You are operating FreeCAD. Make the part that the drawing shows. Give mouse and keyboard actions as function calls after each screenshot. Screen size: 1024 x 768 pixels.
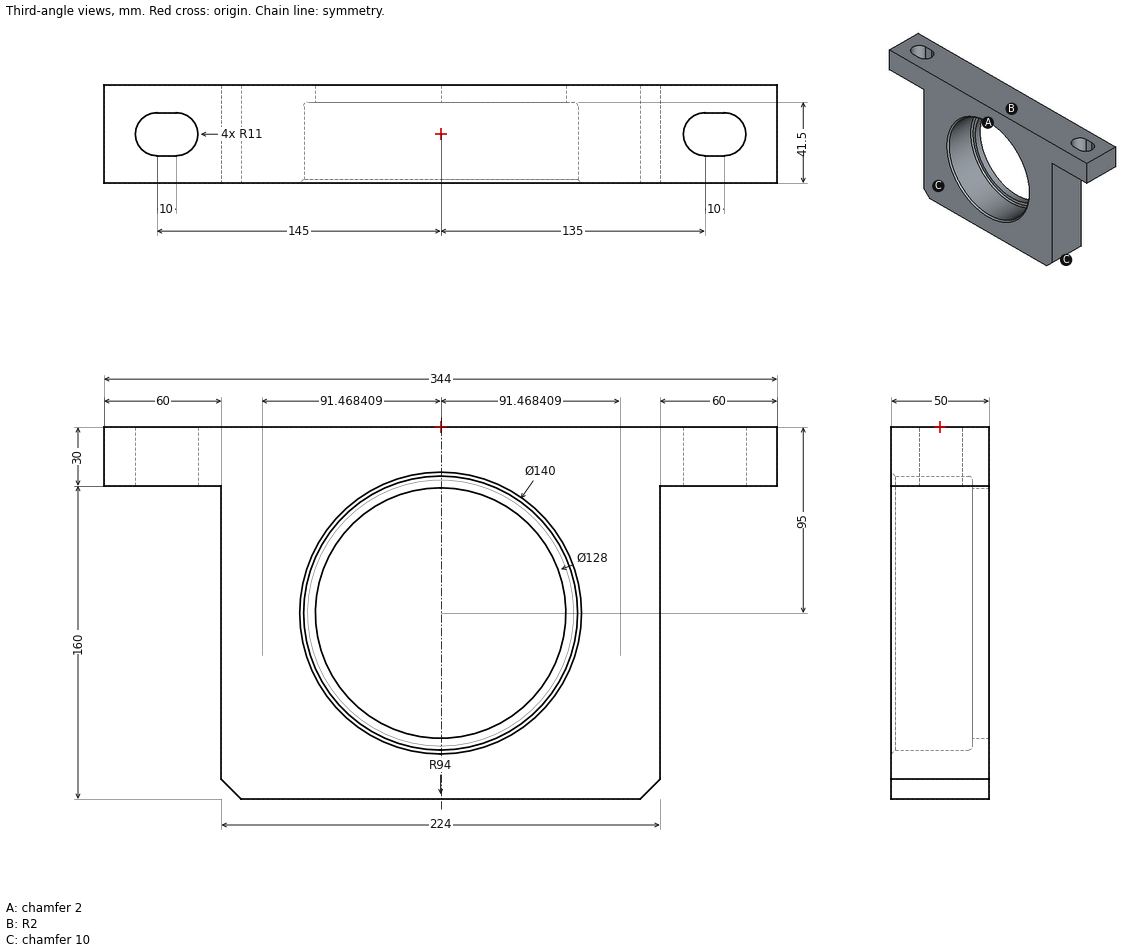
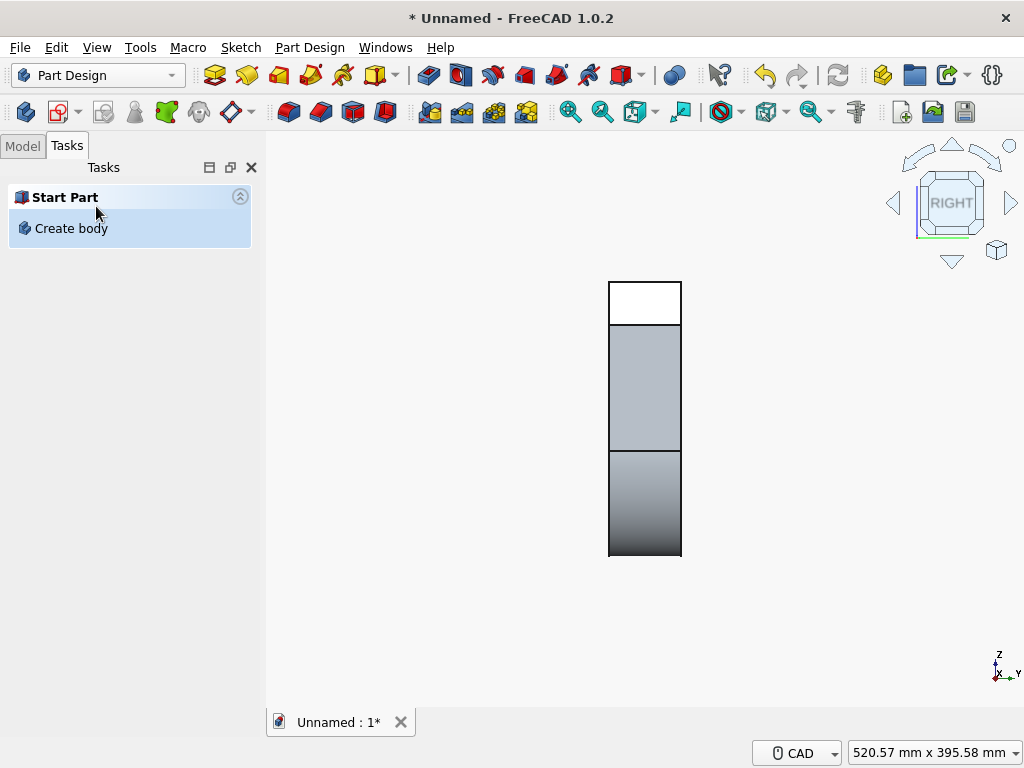
key(5)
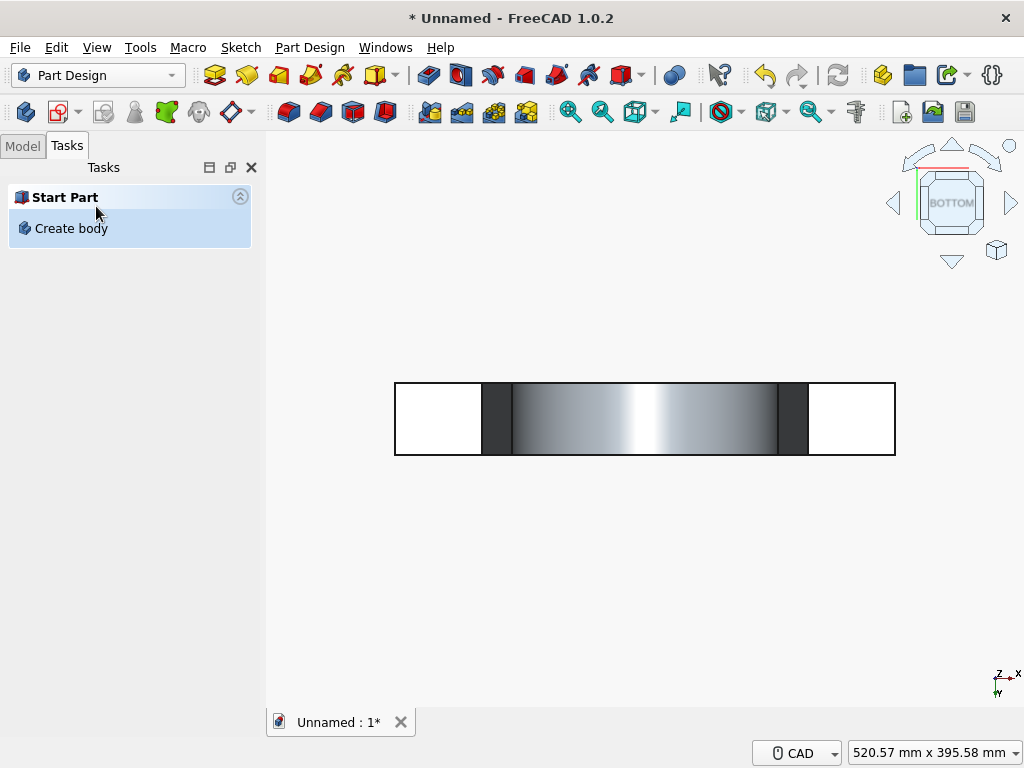
key(4)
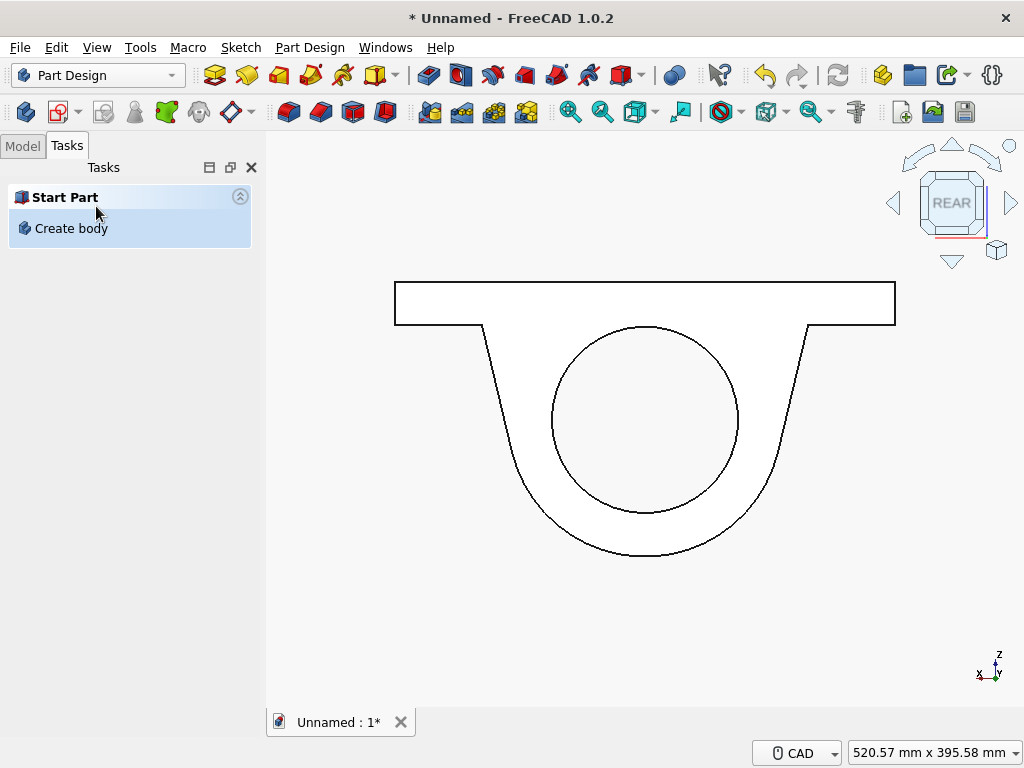
key(6)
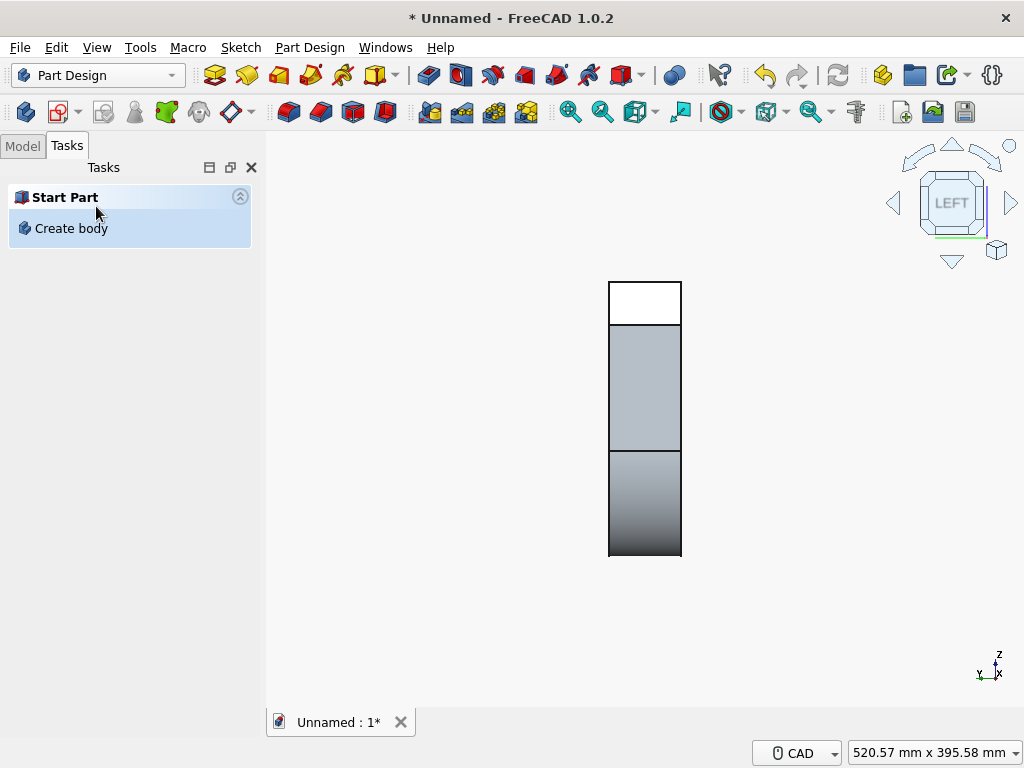
key(v)
key(3)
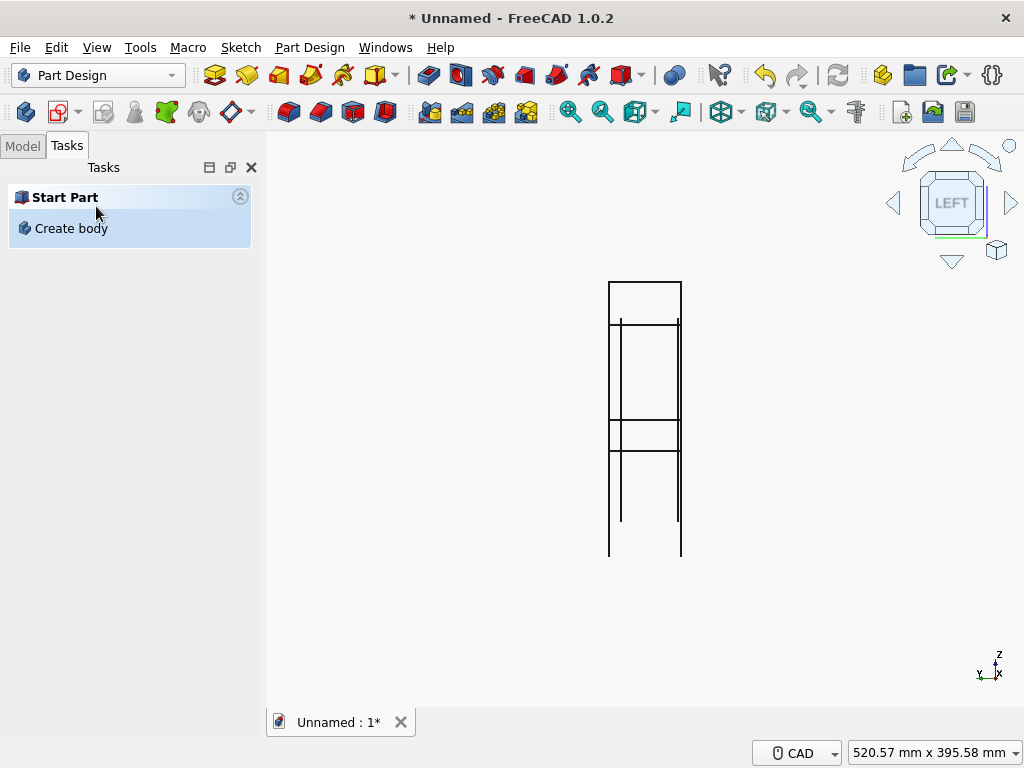
key(0)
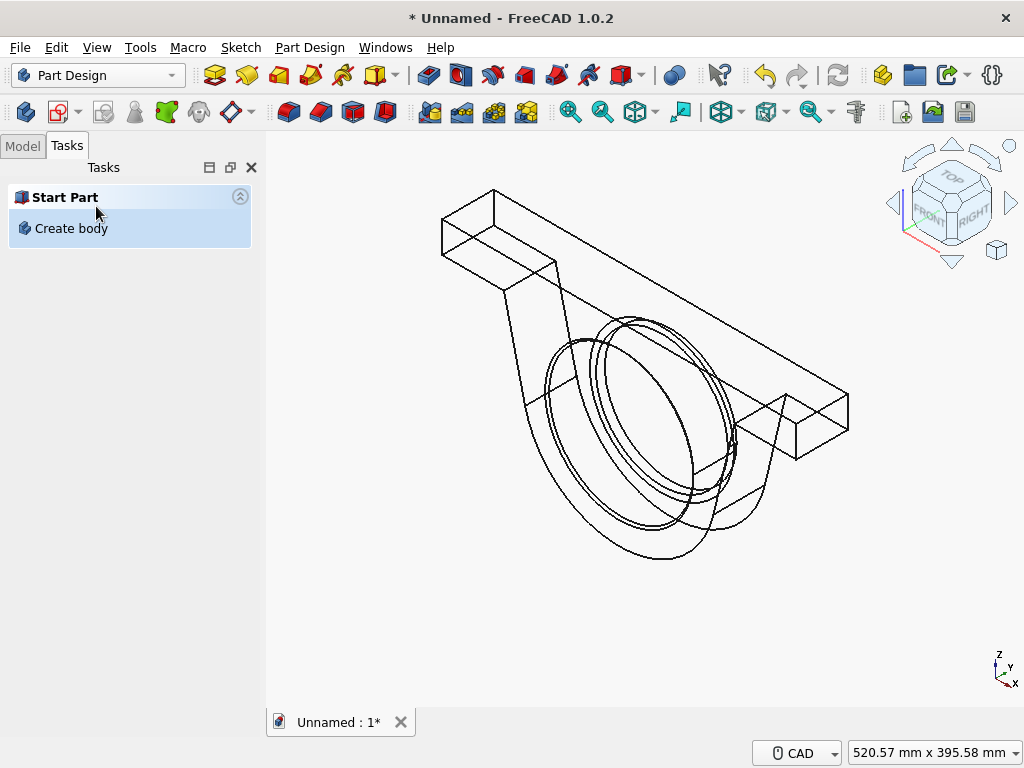
click(590, 367)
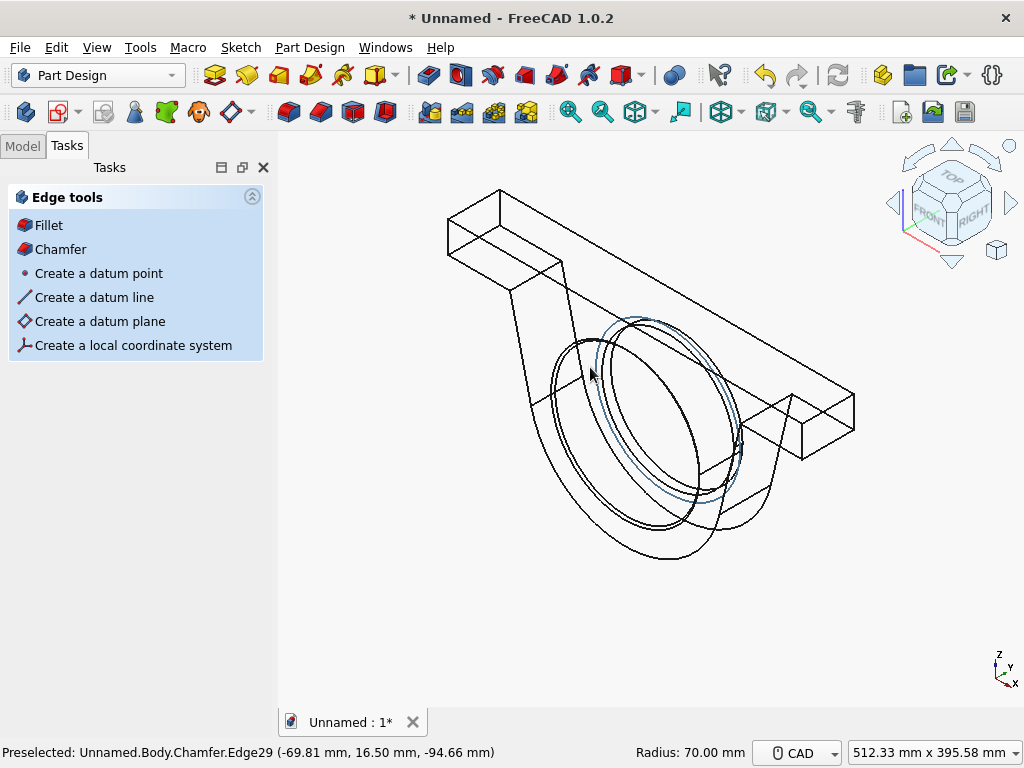
key(v)
key(1)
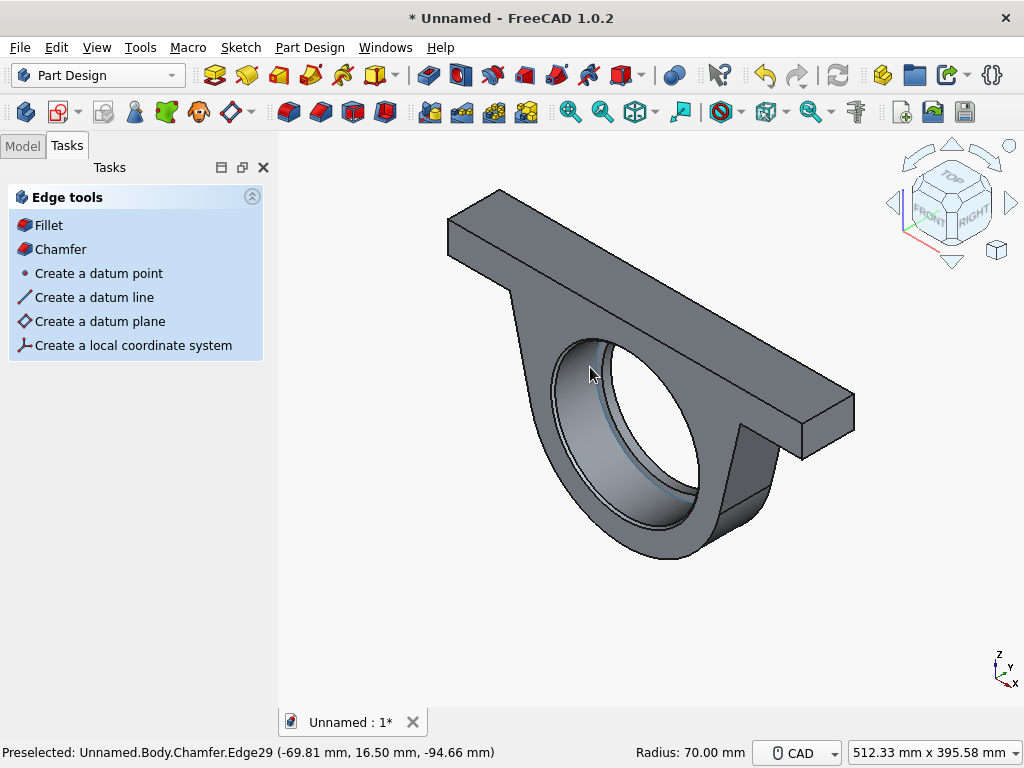
click(290, 112)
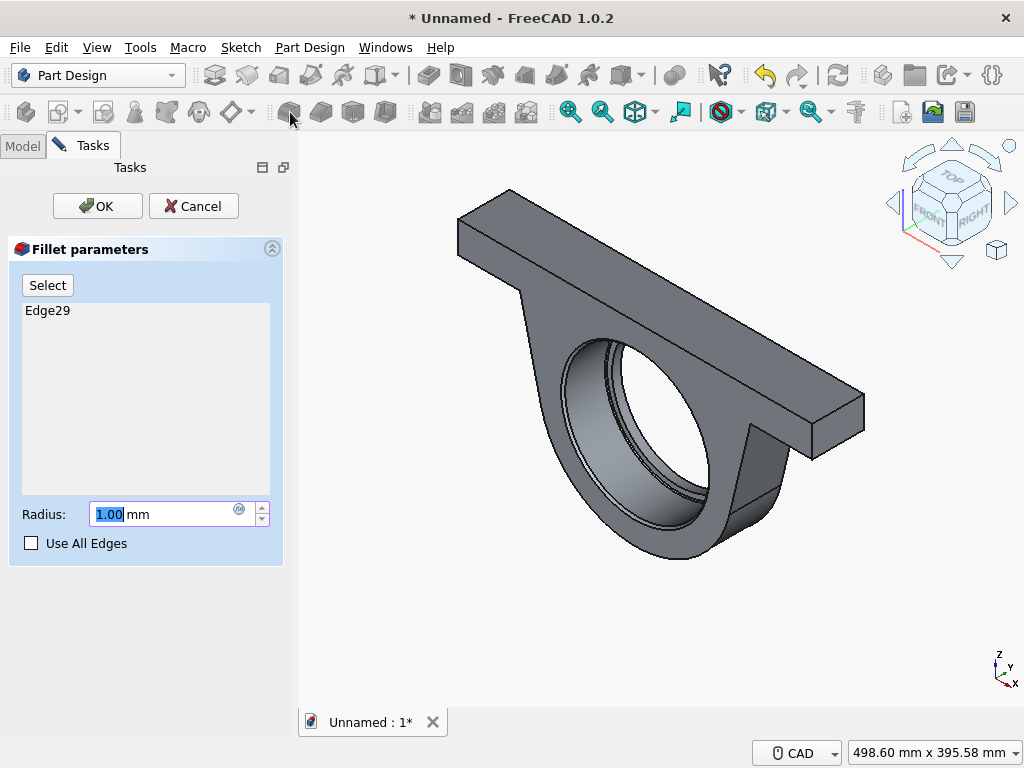
text(2)
key(Tab)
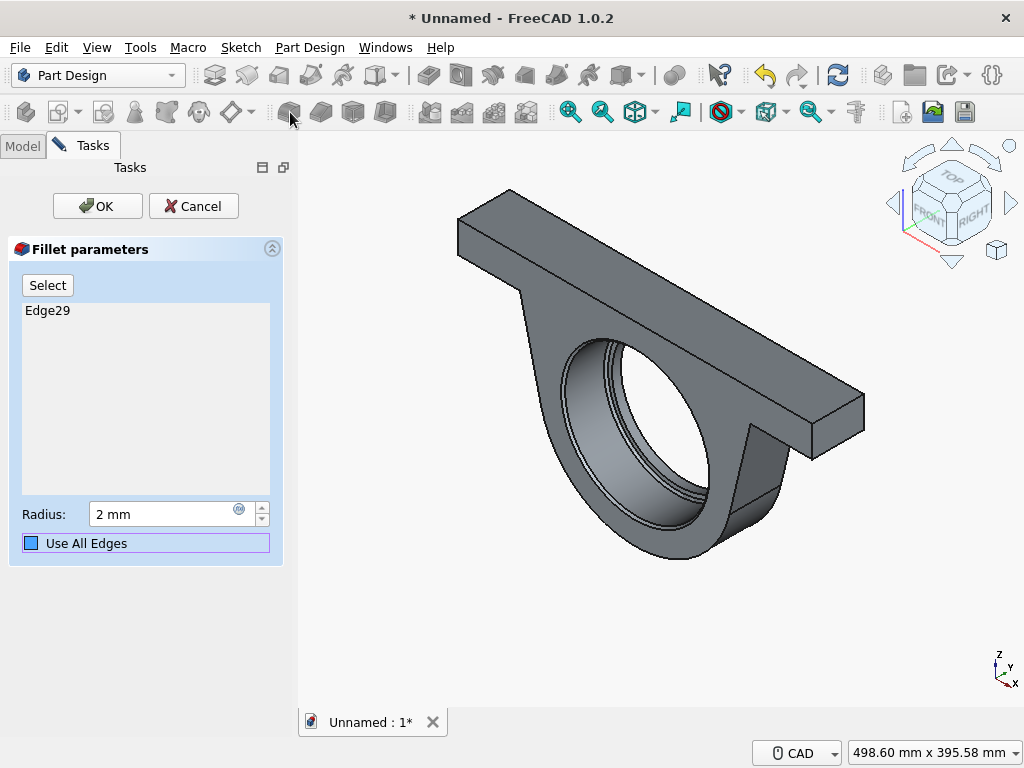
click(98, 206)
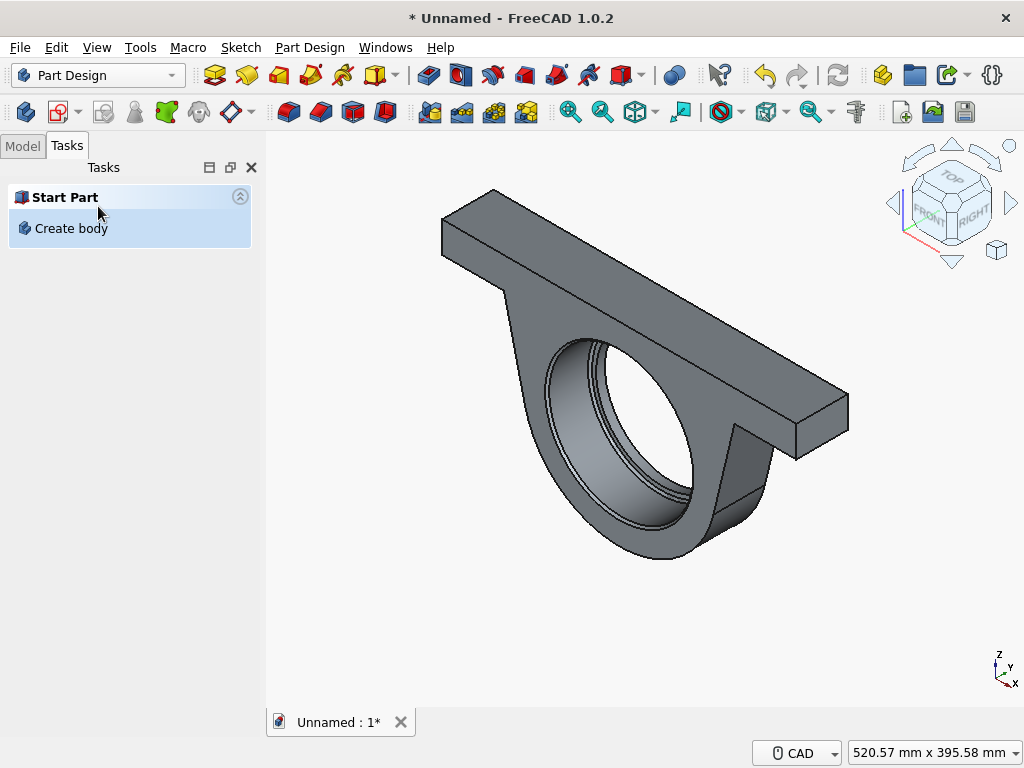
key(5)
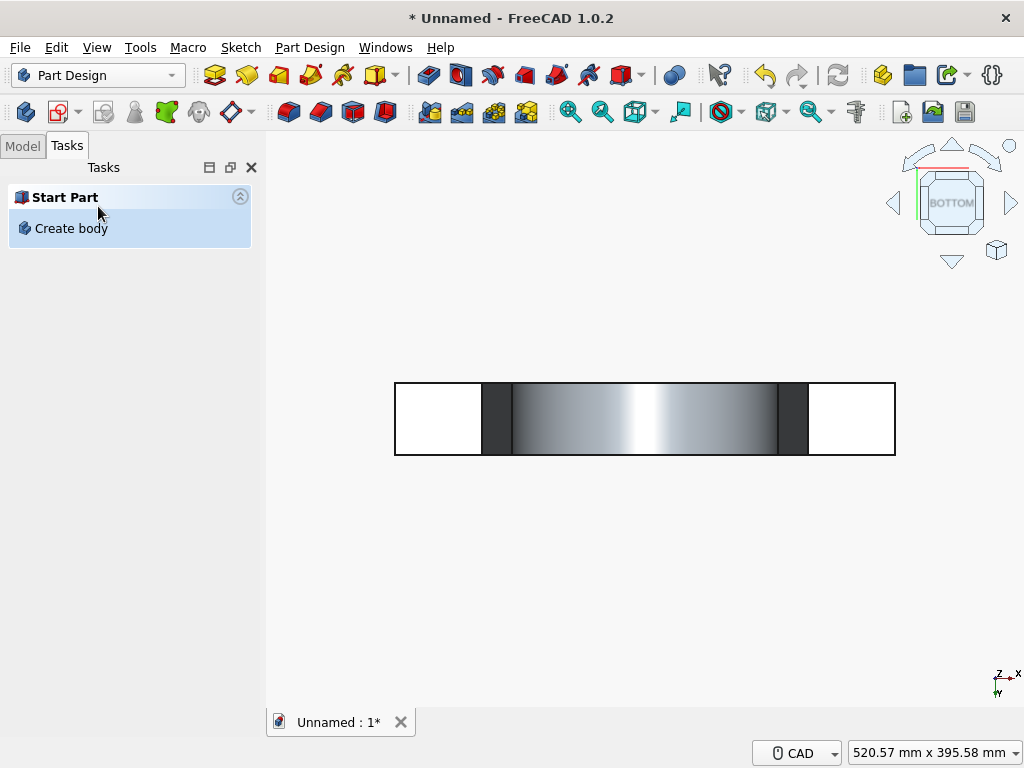
click(438, 418)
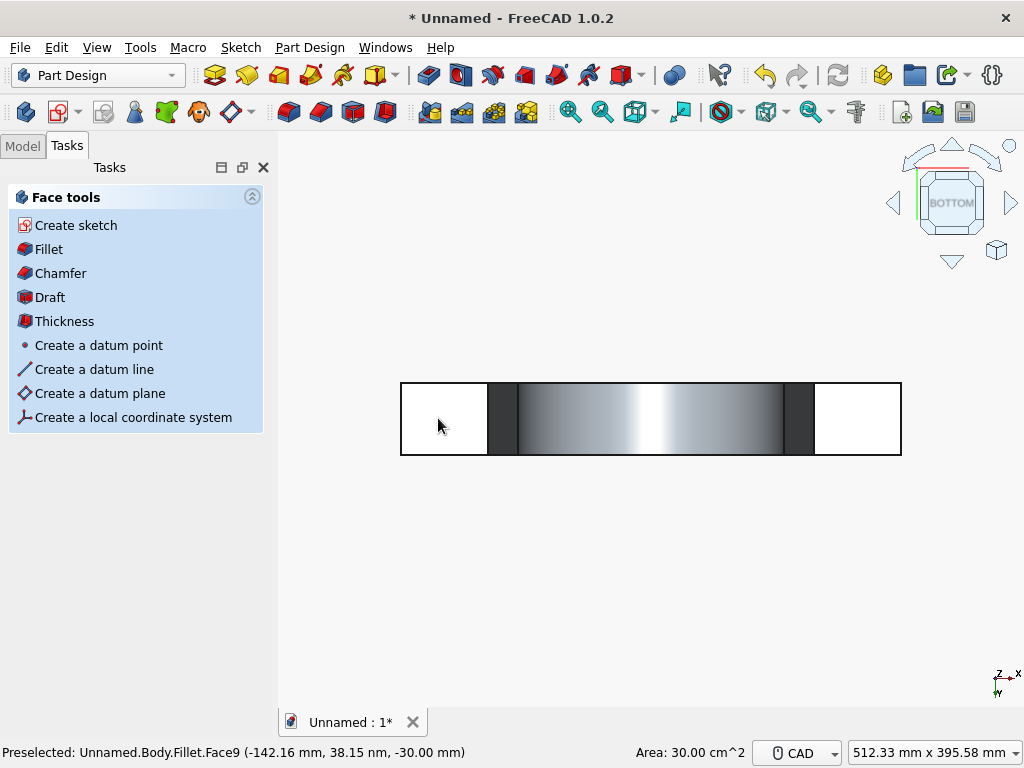
click(58, 112)